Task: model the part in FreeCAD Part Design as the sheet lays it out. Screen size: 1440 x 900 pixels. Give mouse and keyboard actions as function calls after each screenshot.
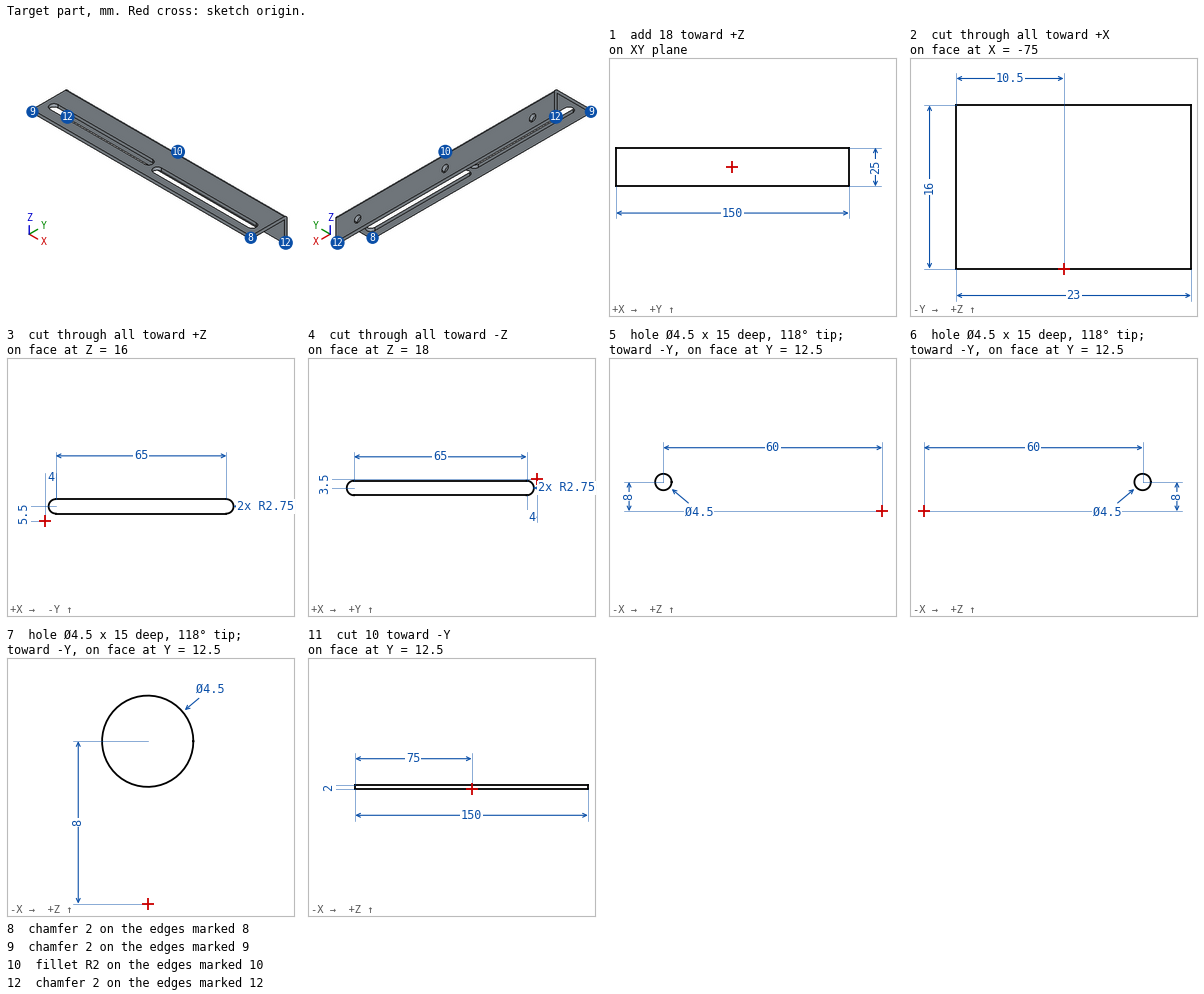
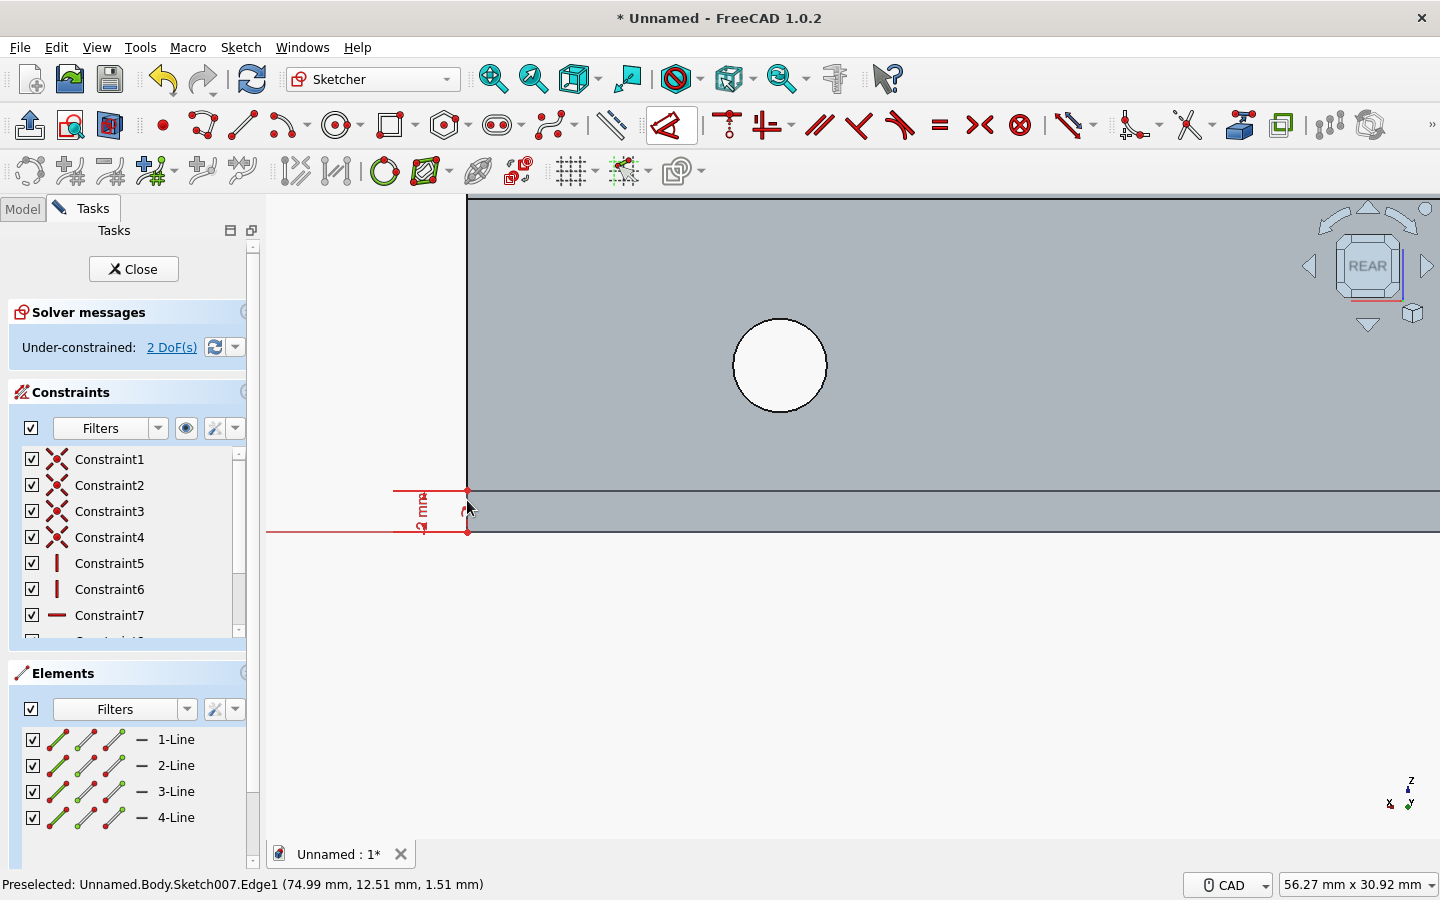
scroll(469, 518, down, 8)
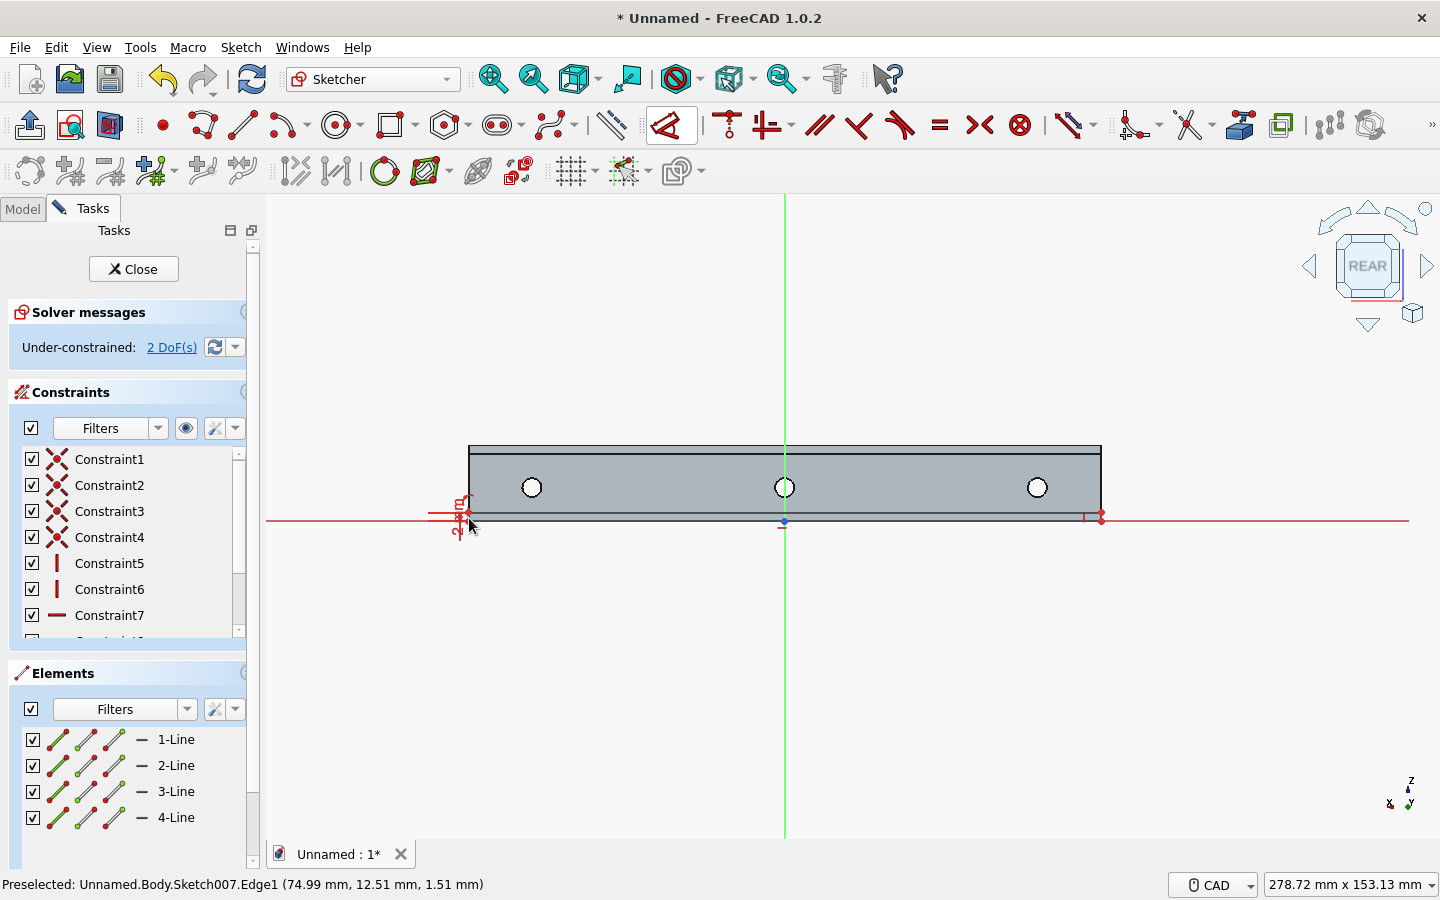
scroll(595, 521, up, 3)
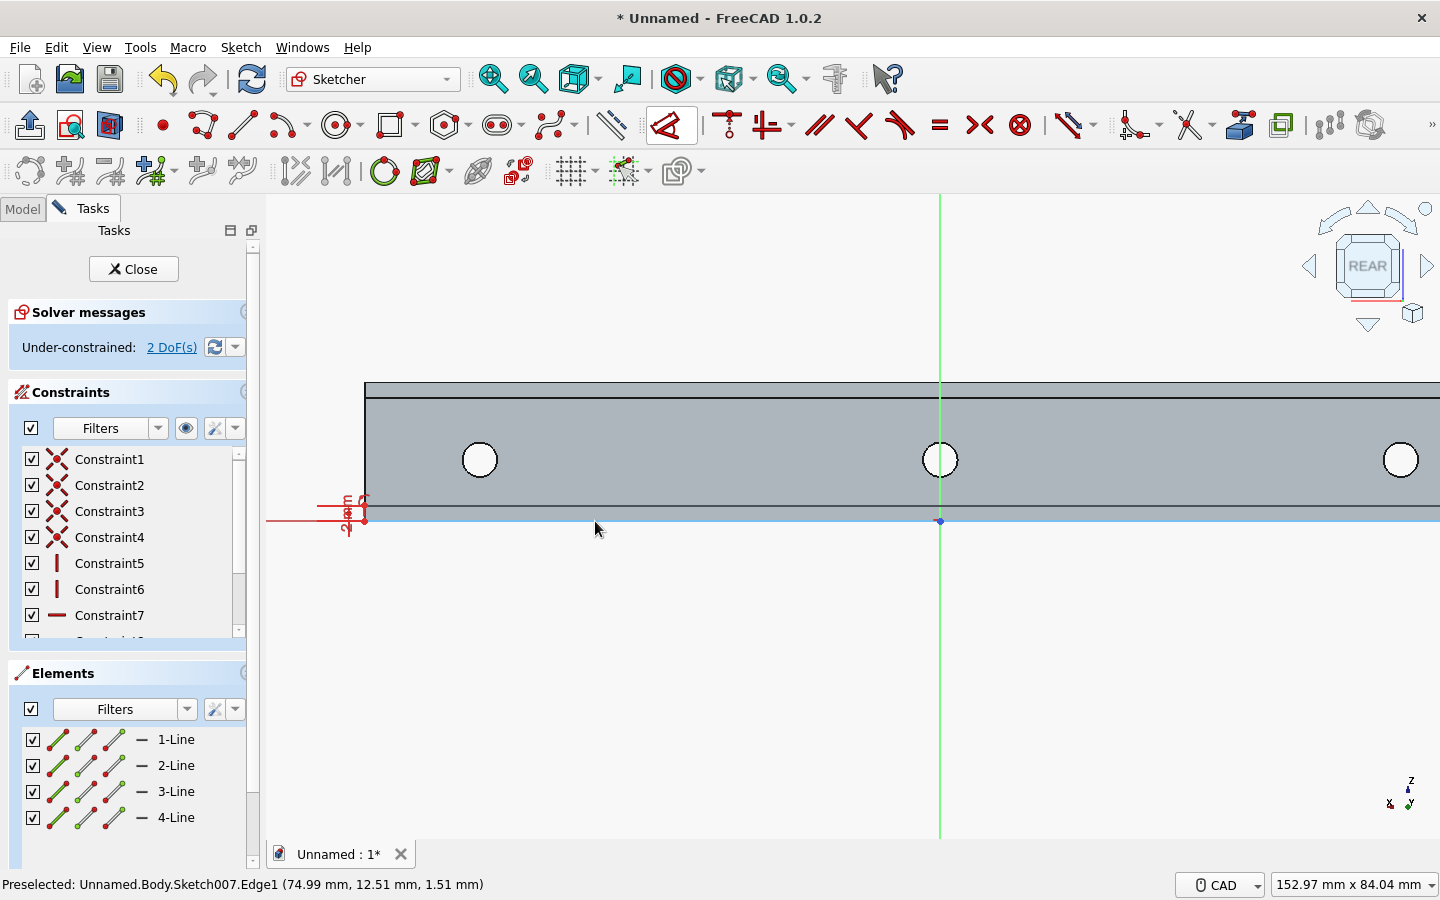
click(595, 521)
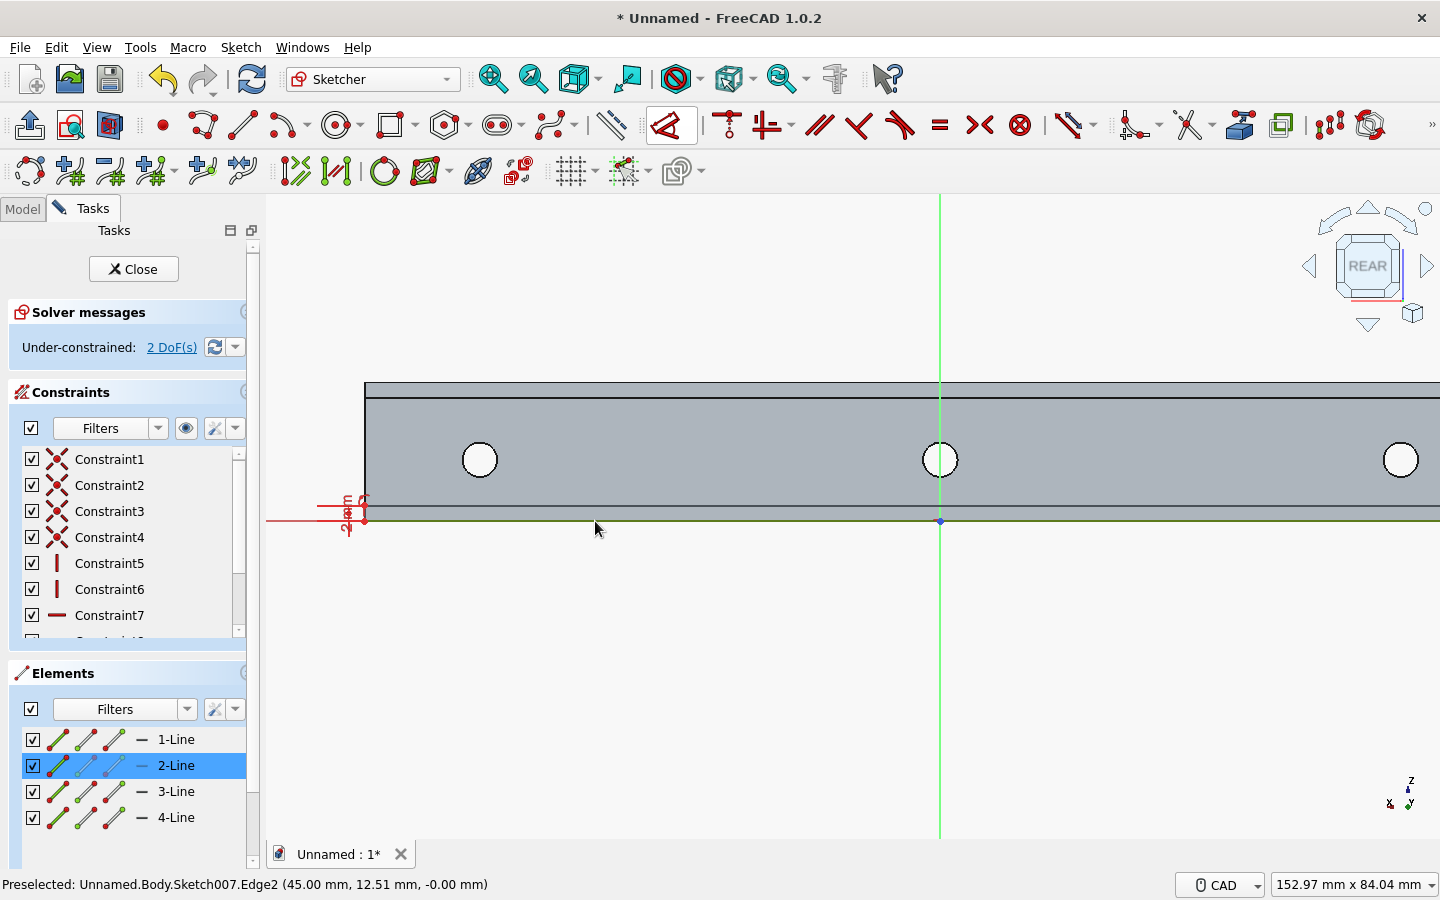
click(692, 126)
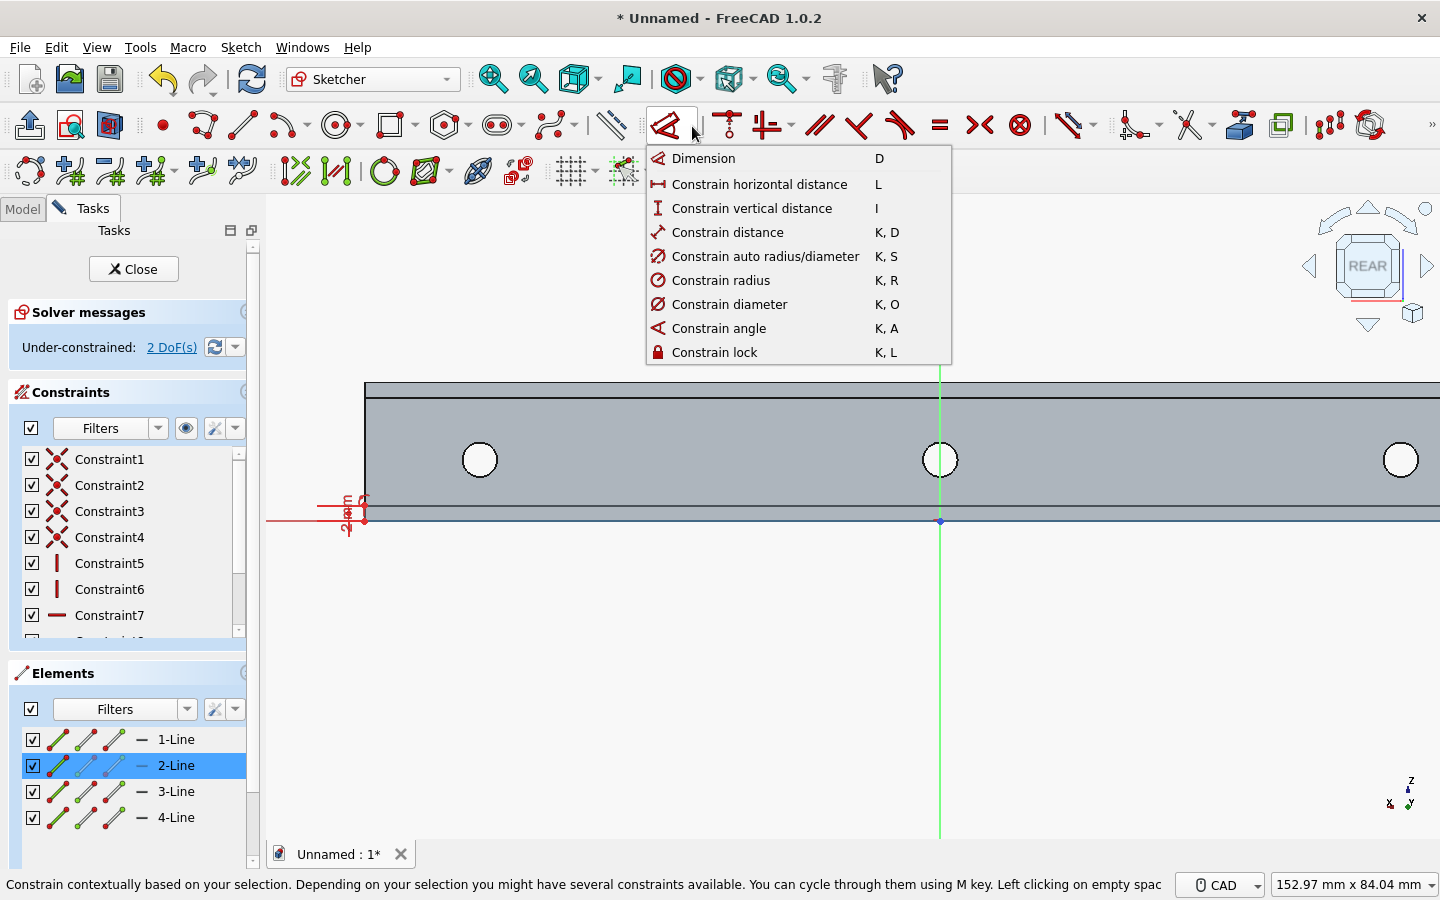
click(799, 184)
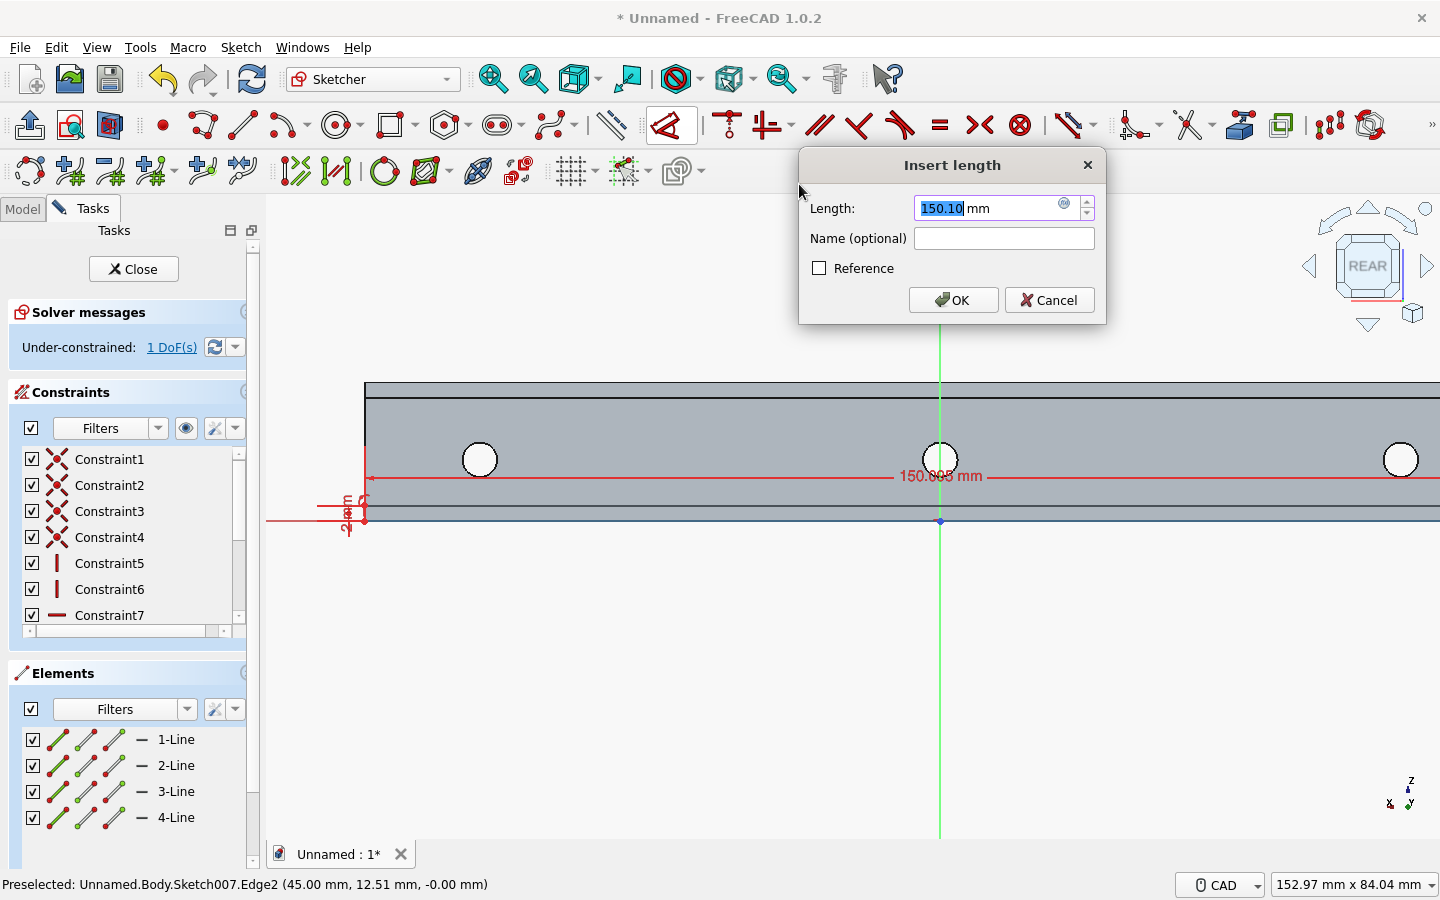
text(150)
key(Return)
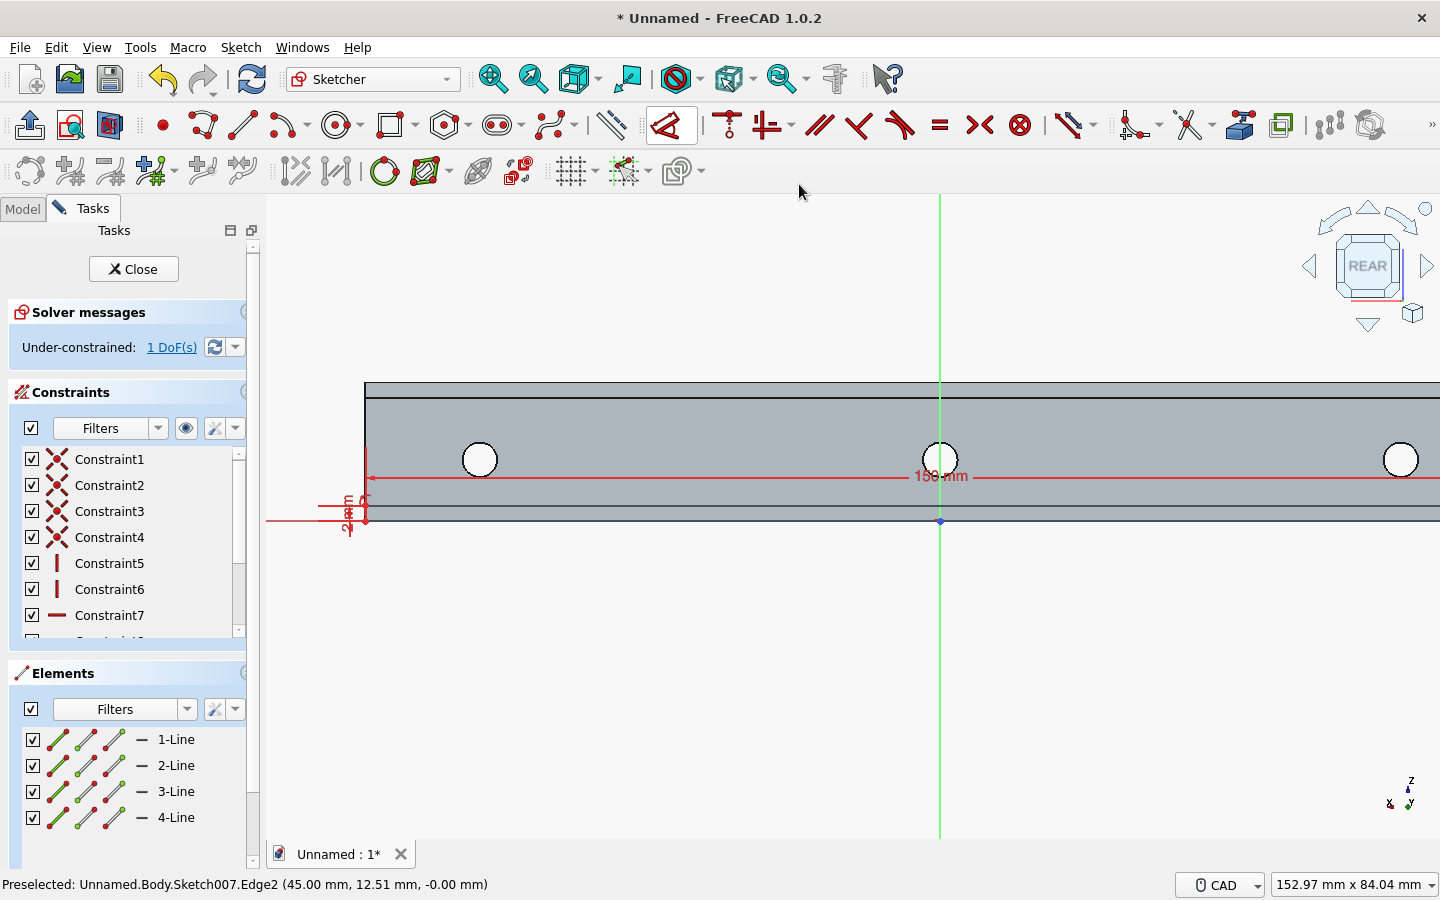
click(366, 506)